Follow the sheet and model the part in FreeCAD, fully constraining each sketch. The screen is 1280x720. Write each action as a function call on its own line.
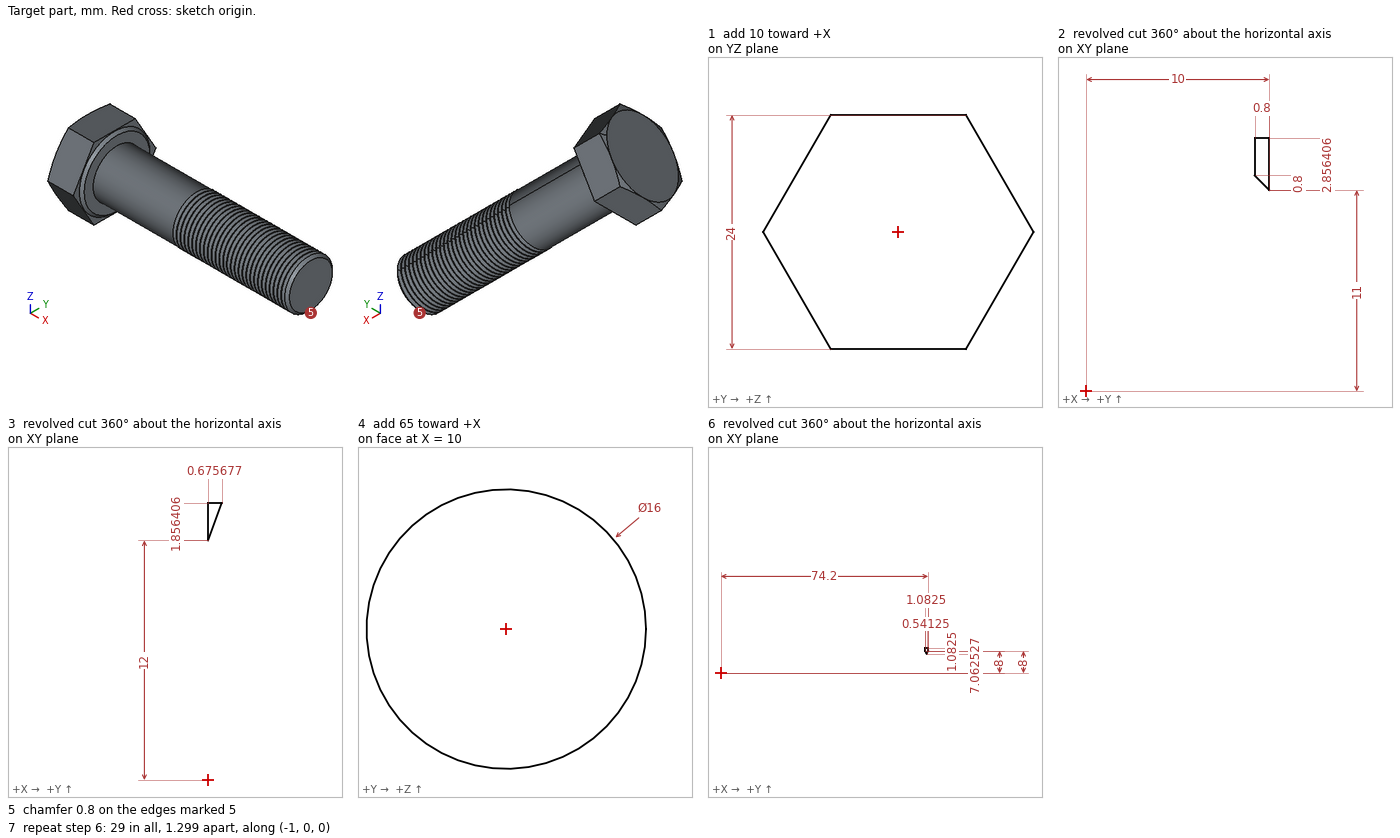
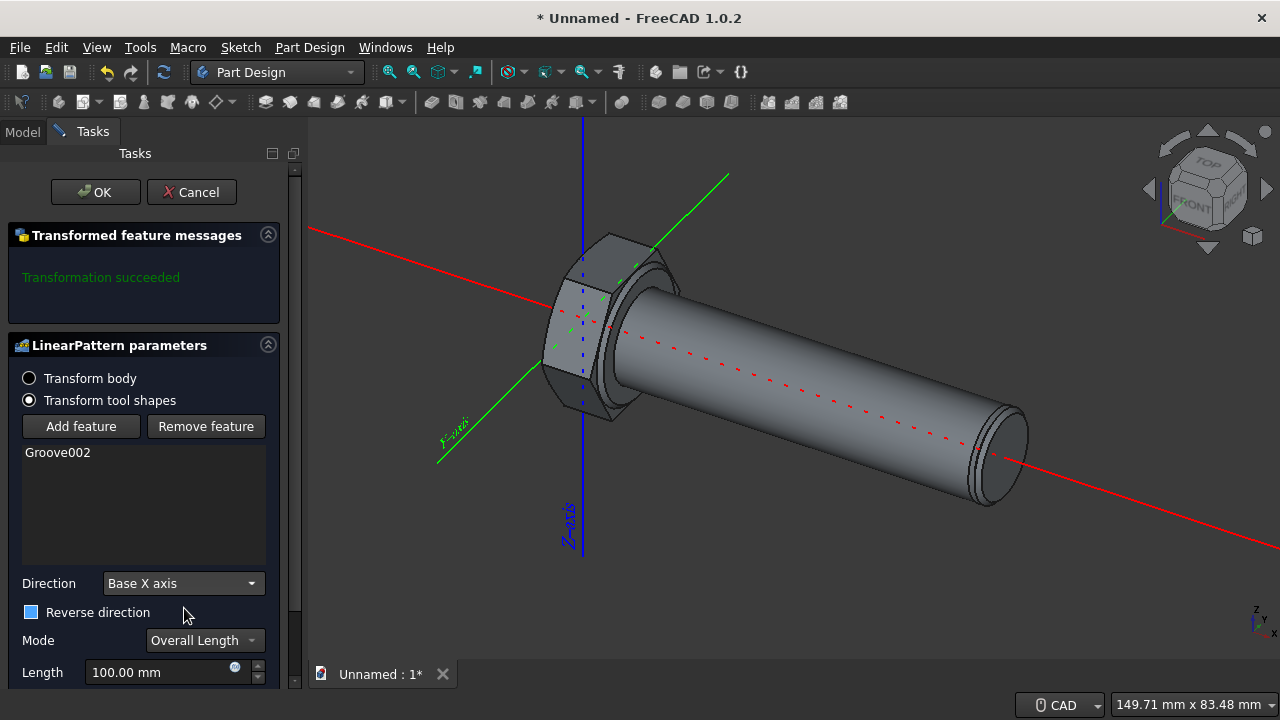
click(206, 640)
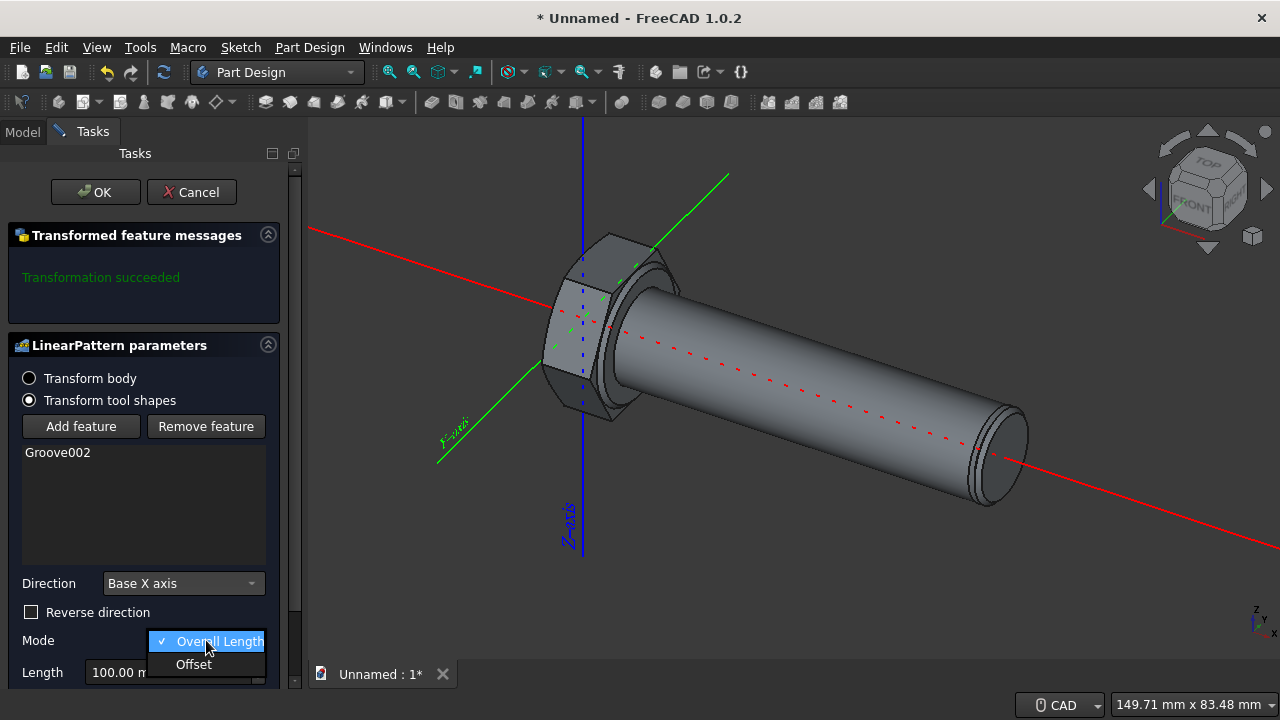
click(206, 664)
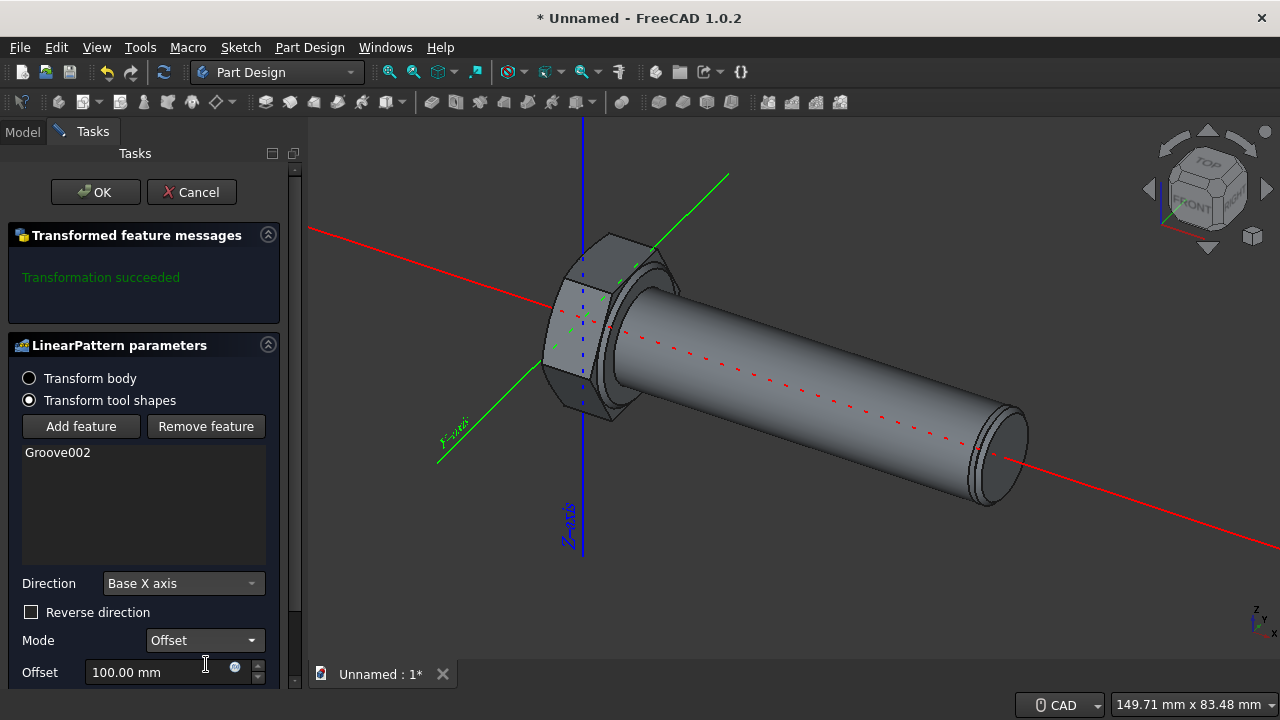
triple_click(168, 672)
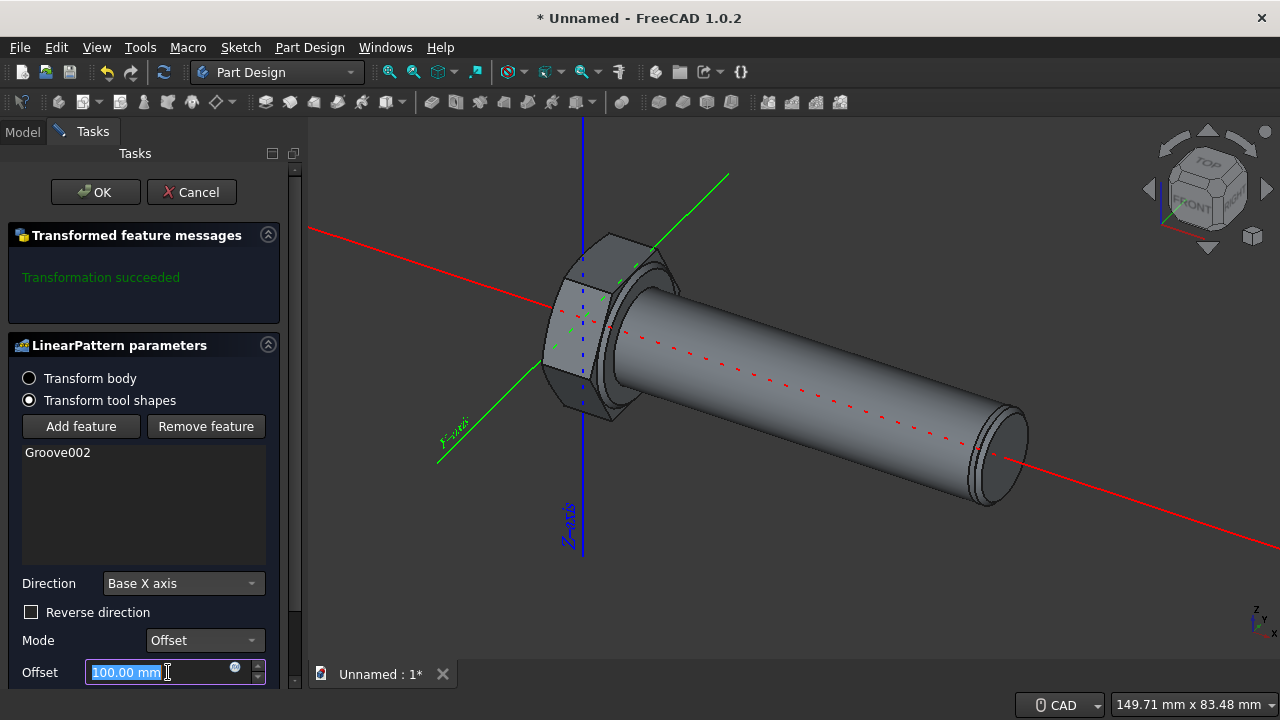
text(1.299)
key(Tab)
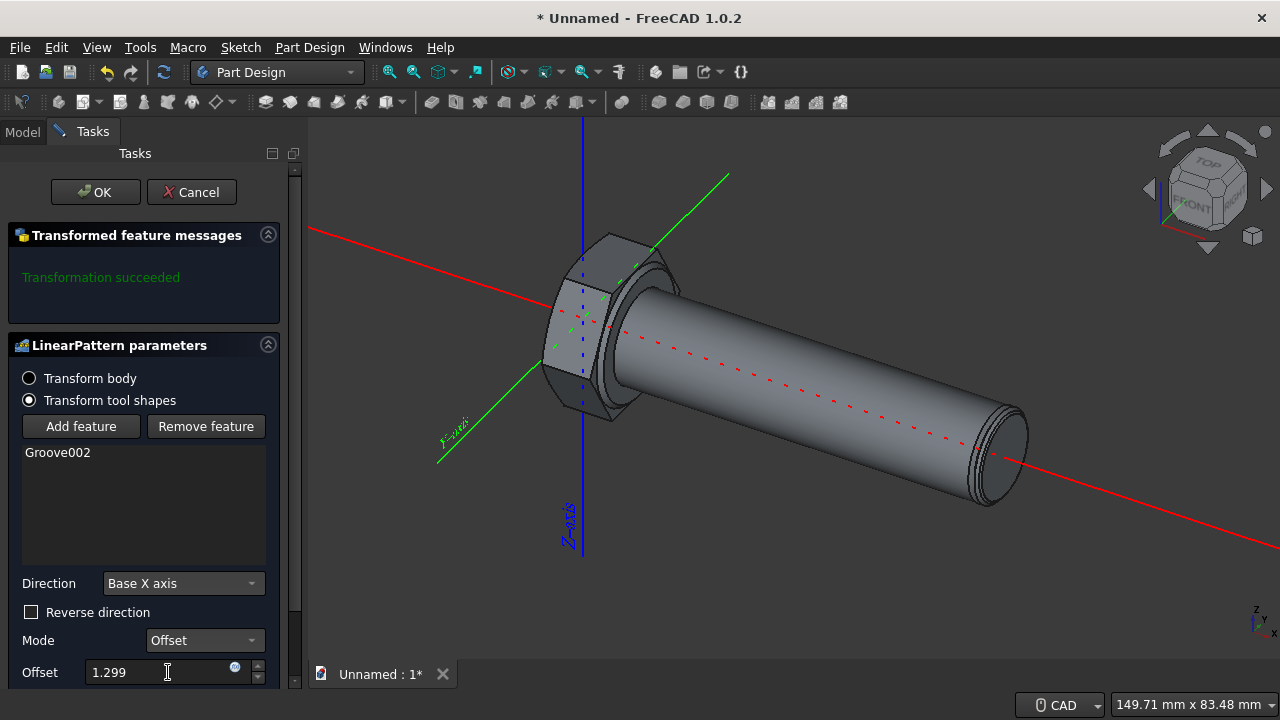
scroll(295, 426, down, 2)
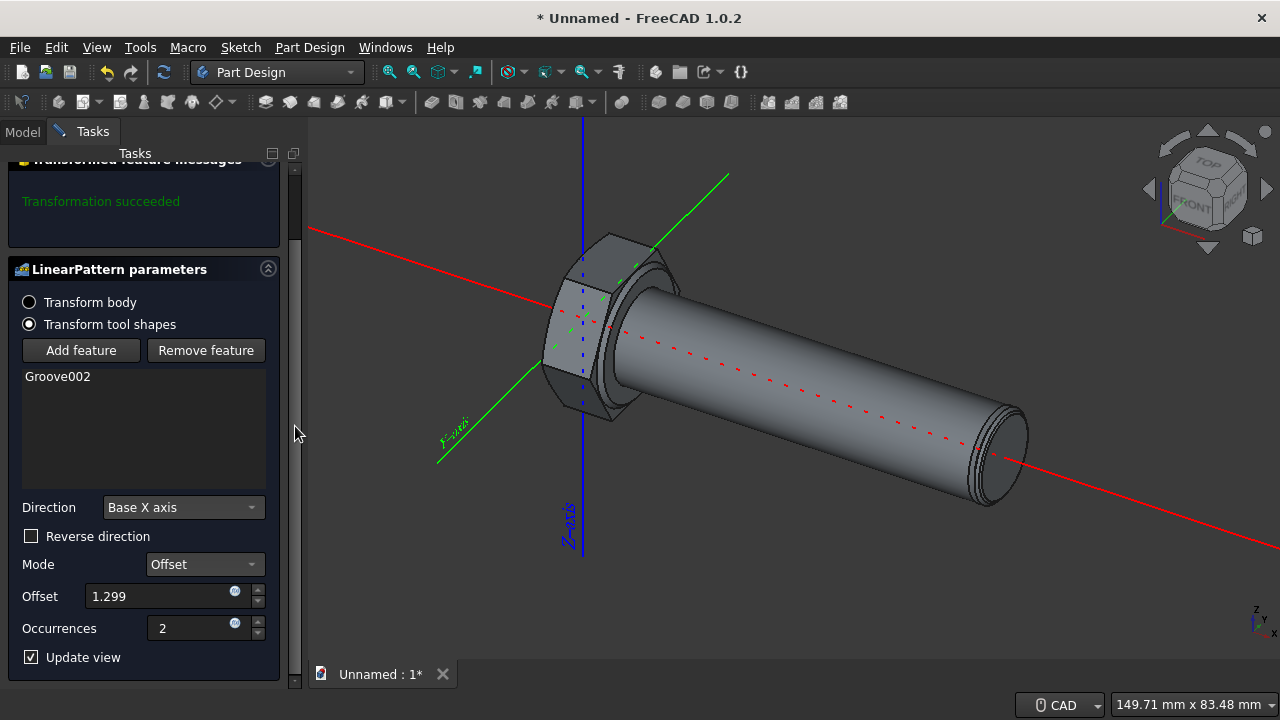
triple_click(198, 628)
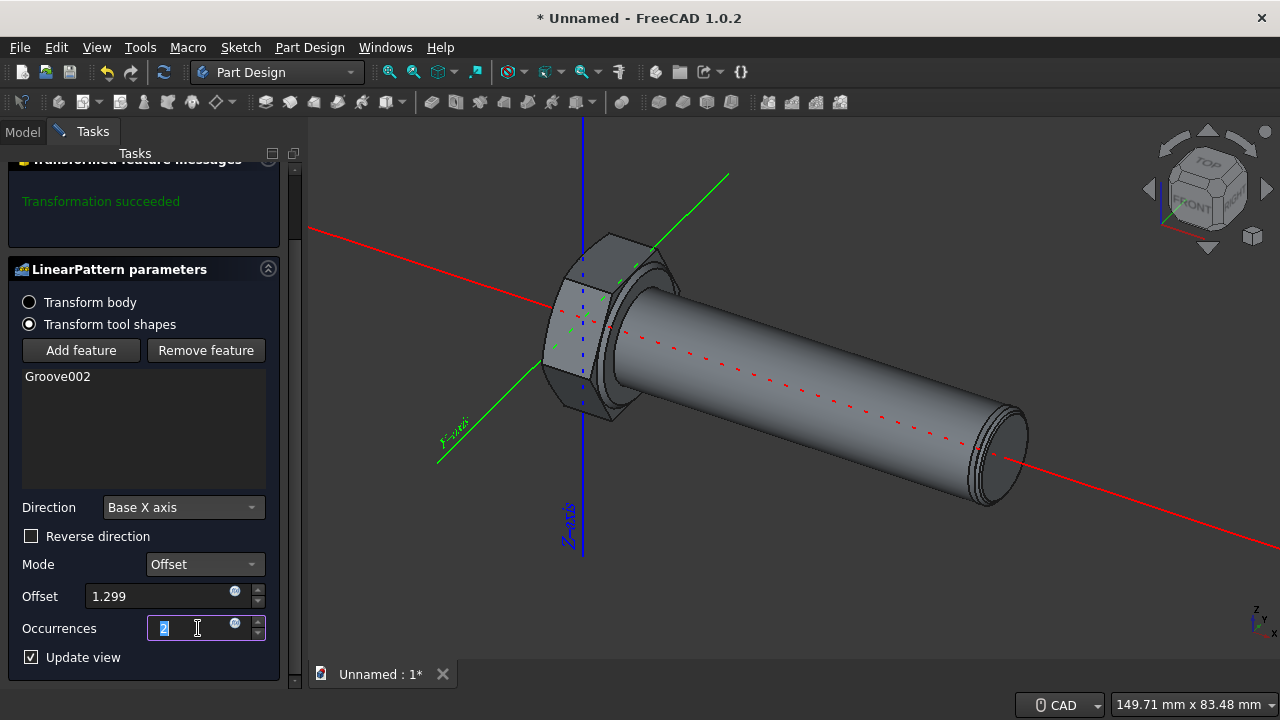
text(29)
key(Tab)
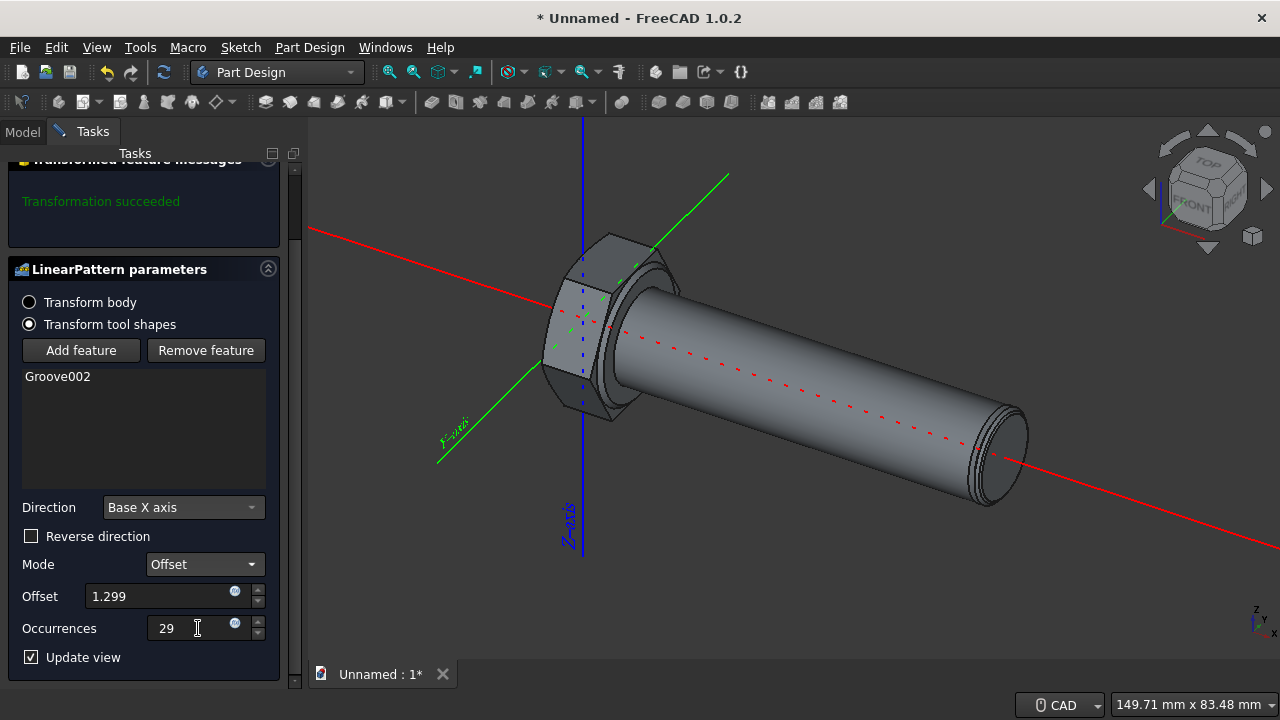
click(30, 536)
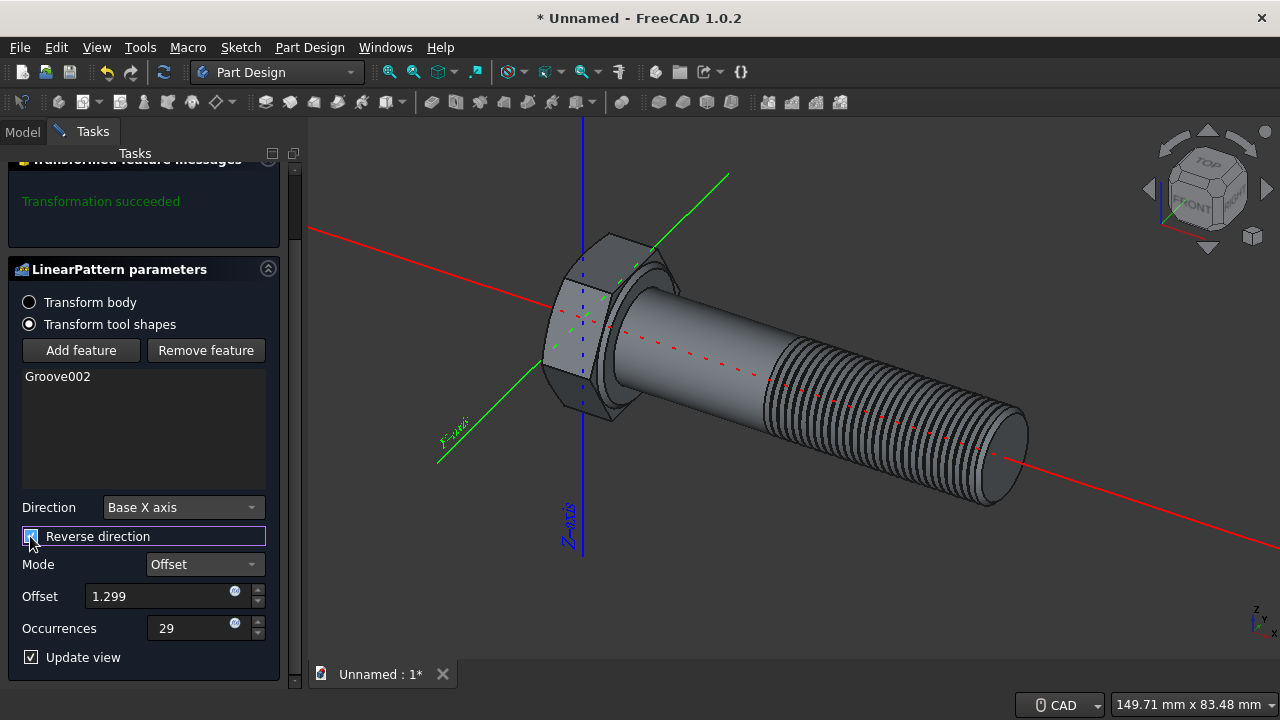
scroll(295, 426, up, 3)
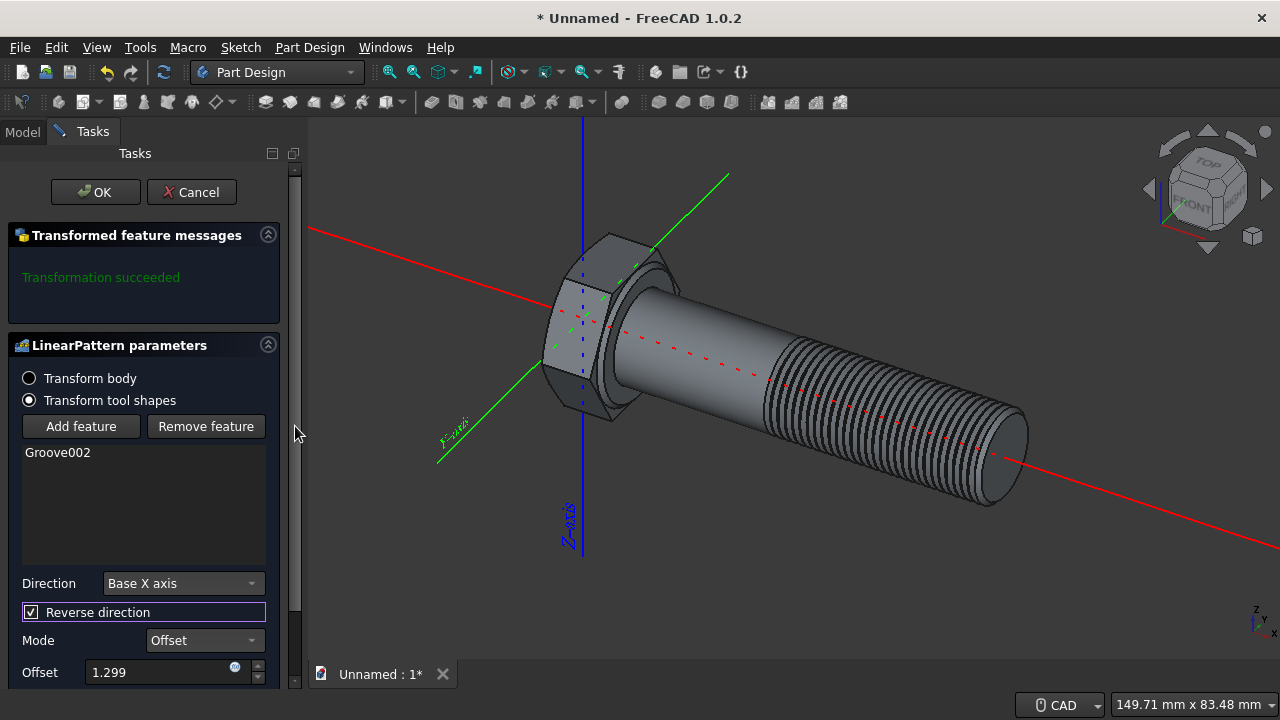
click(96, 192)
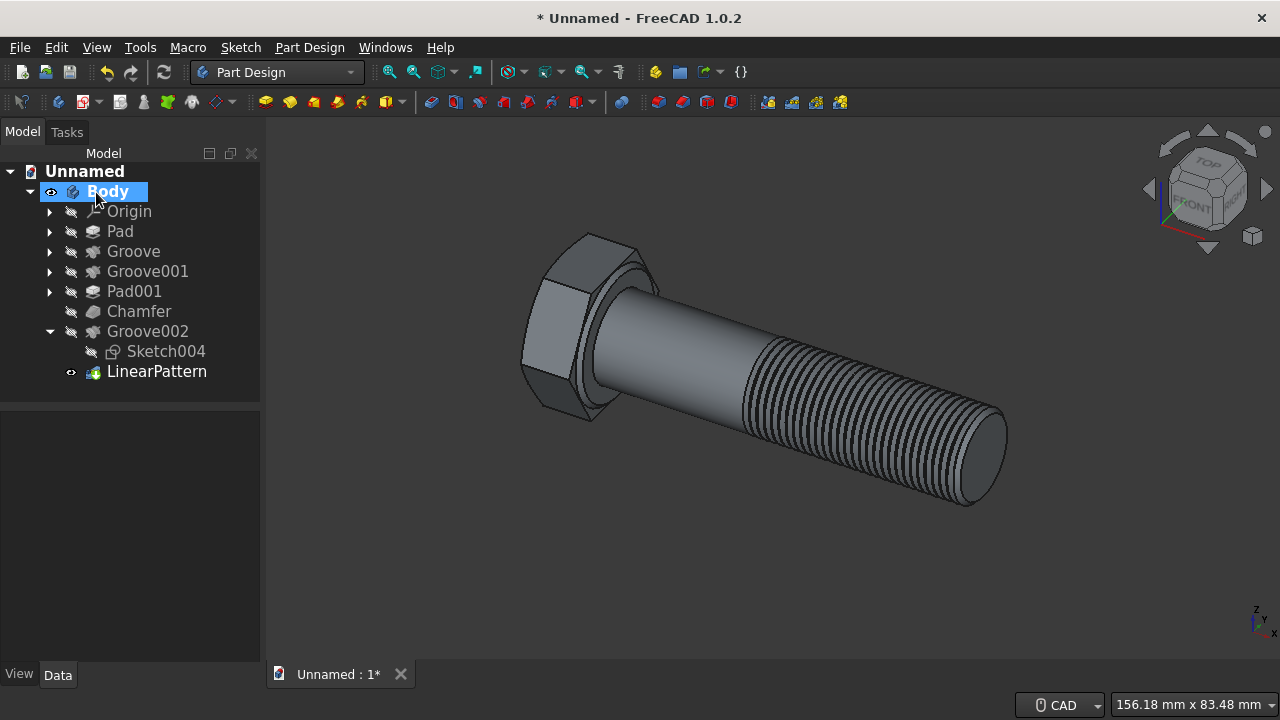
key(0)